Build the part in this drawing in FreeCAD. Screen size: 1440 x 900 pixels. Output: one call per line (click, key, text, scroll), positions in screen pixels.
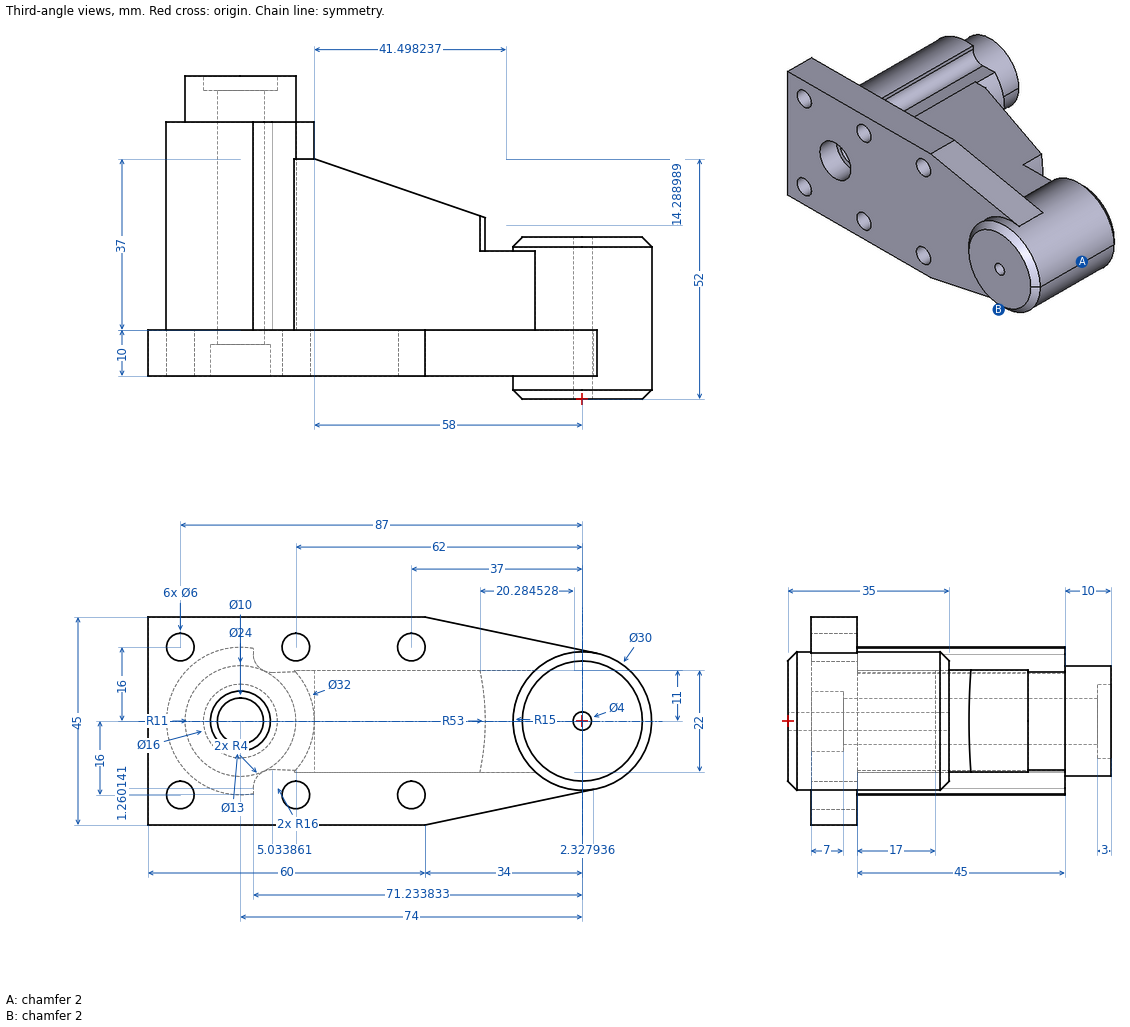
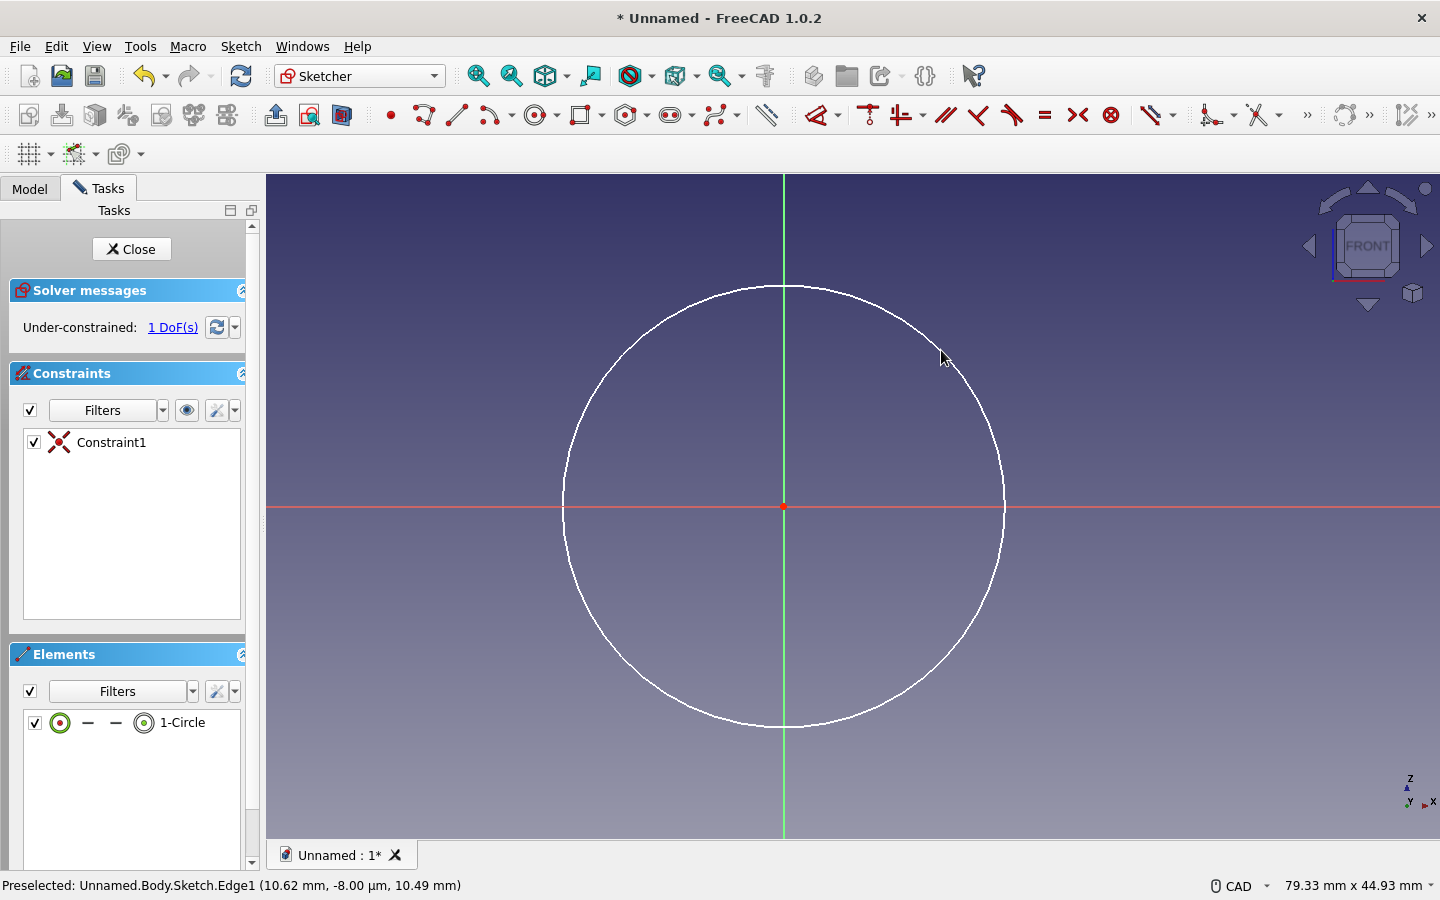
click(940, 350)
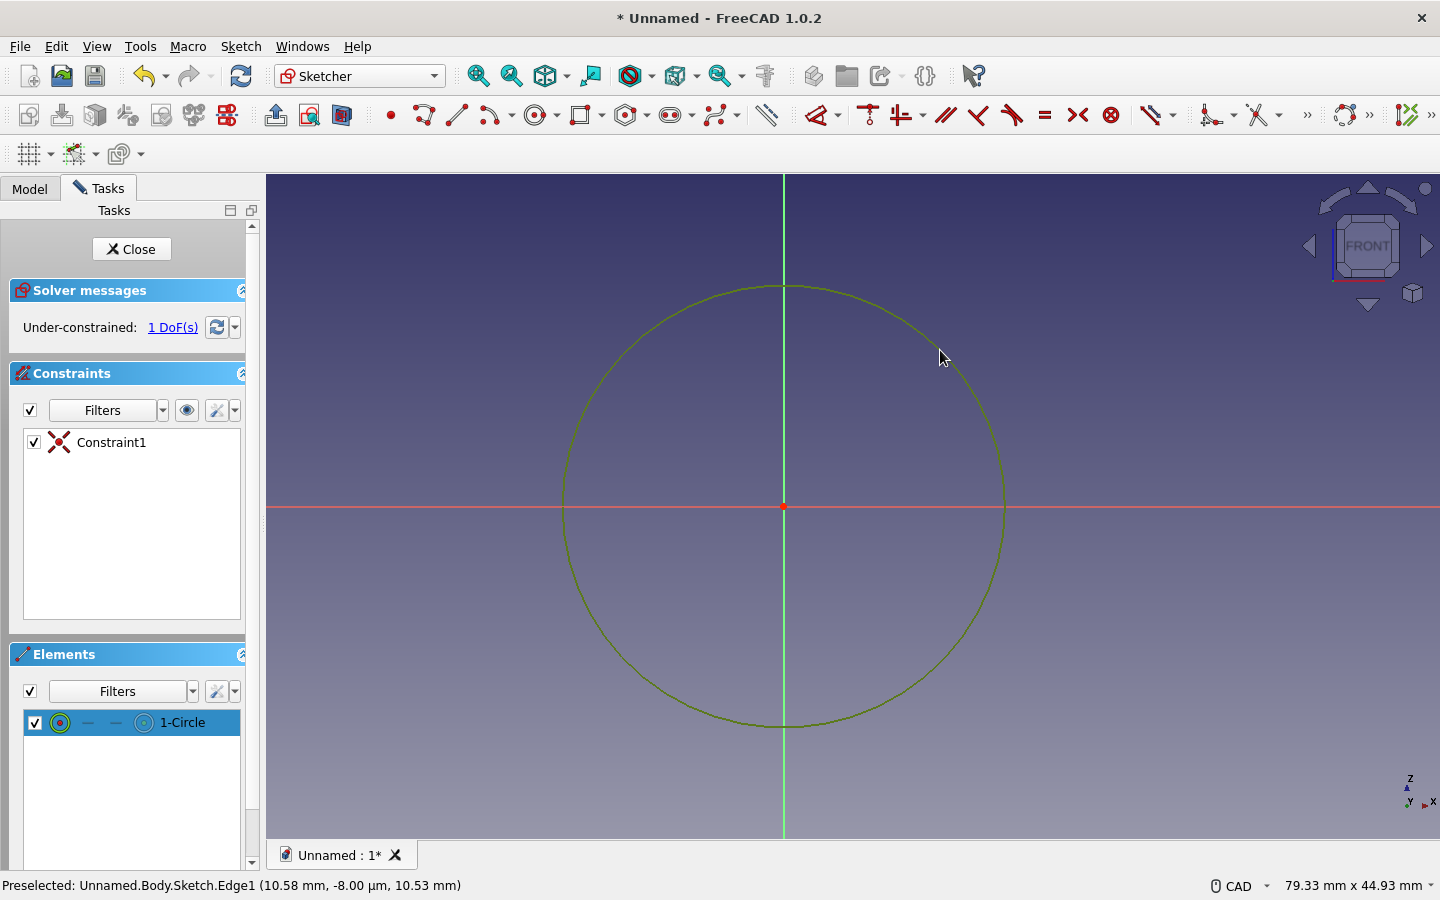
key(k)
key(o)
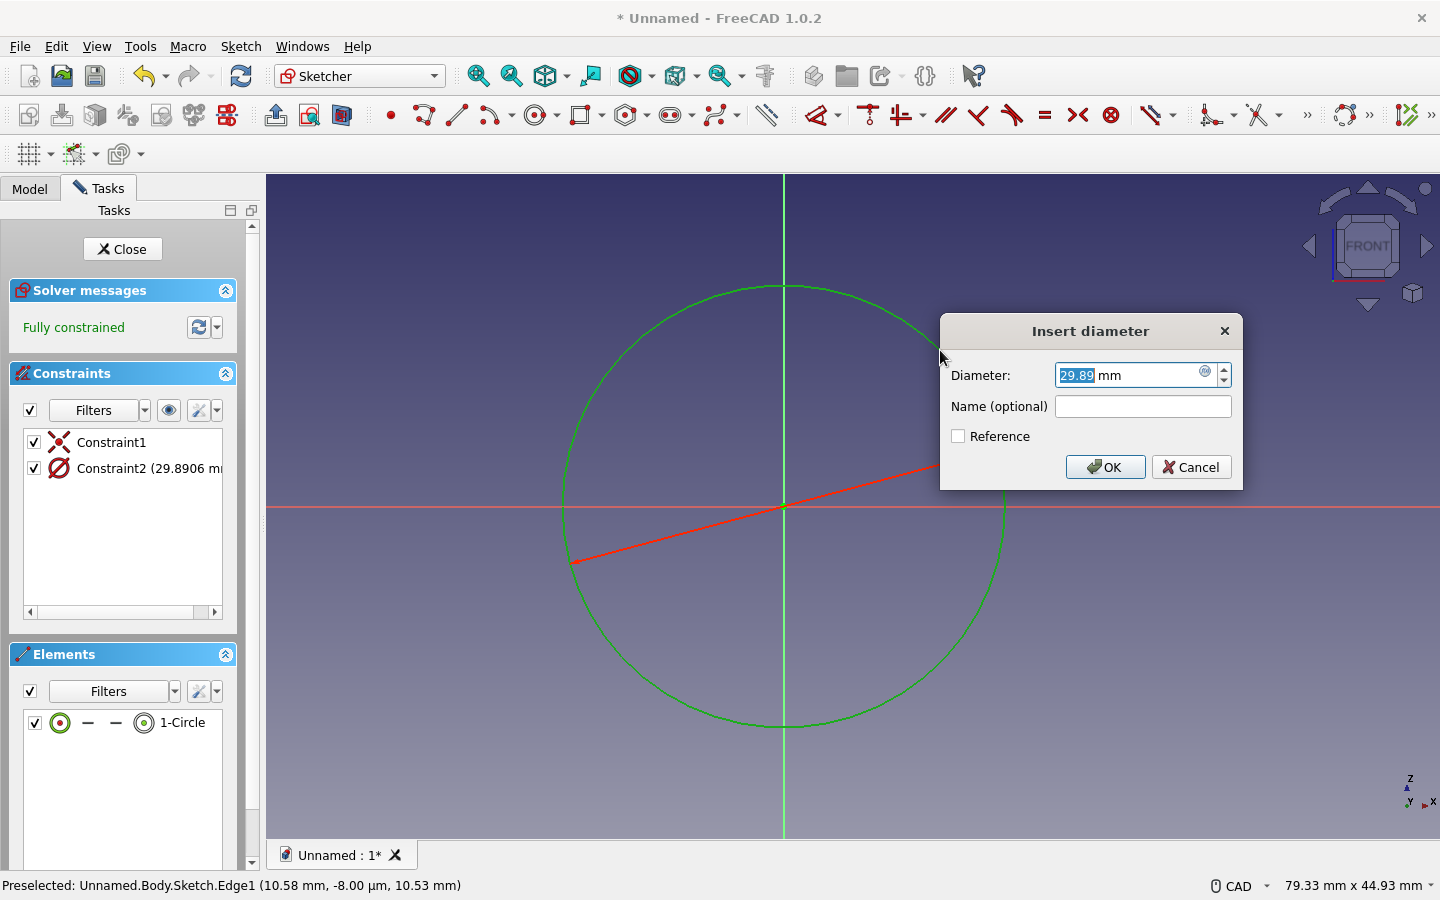
text(30)
key(Return)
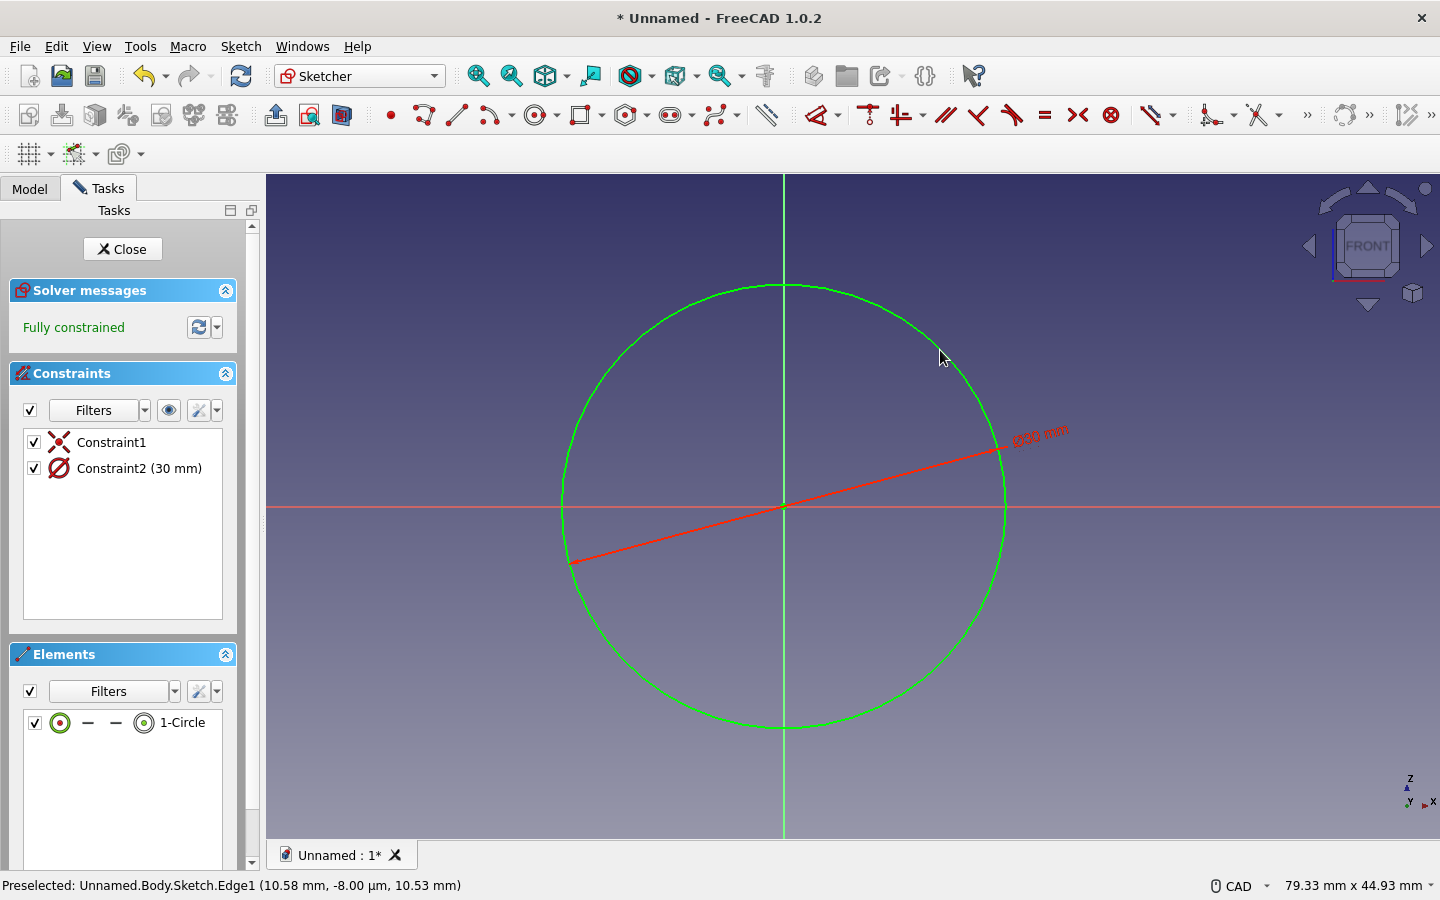
click(123, 249)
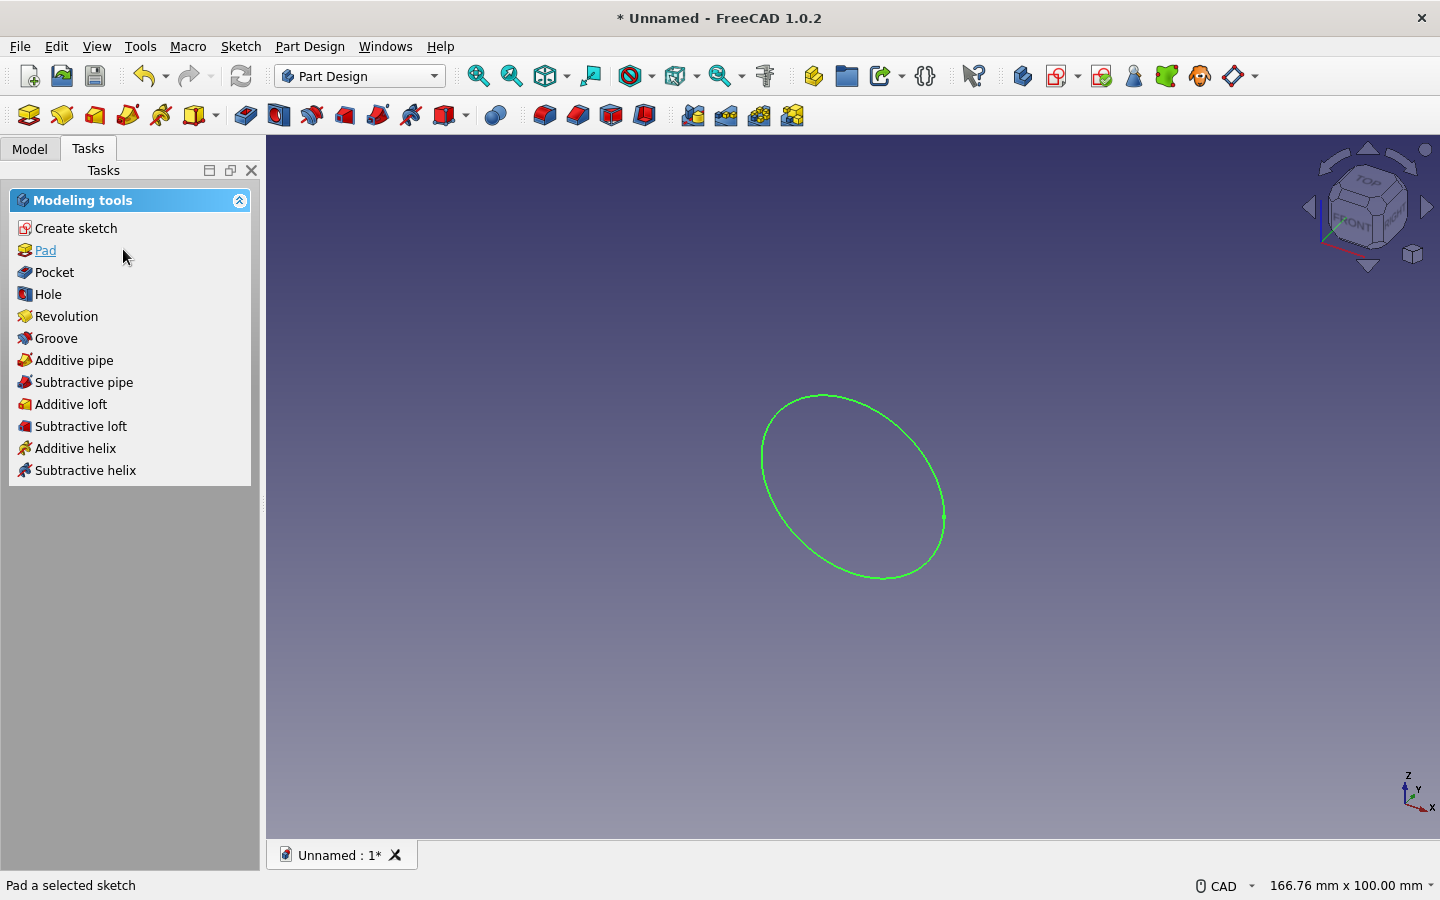
click(29, 116)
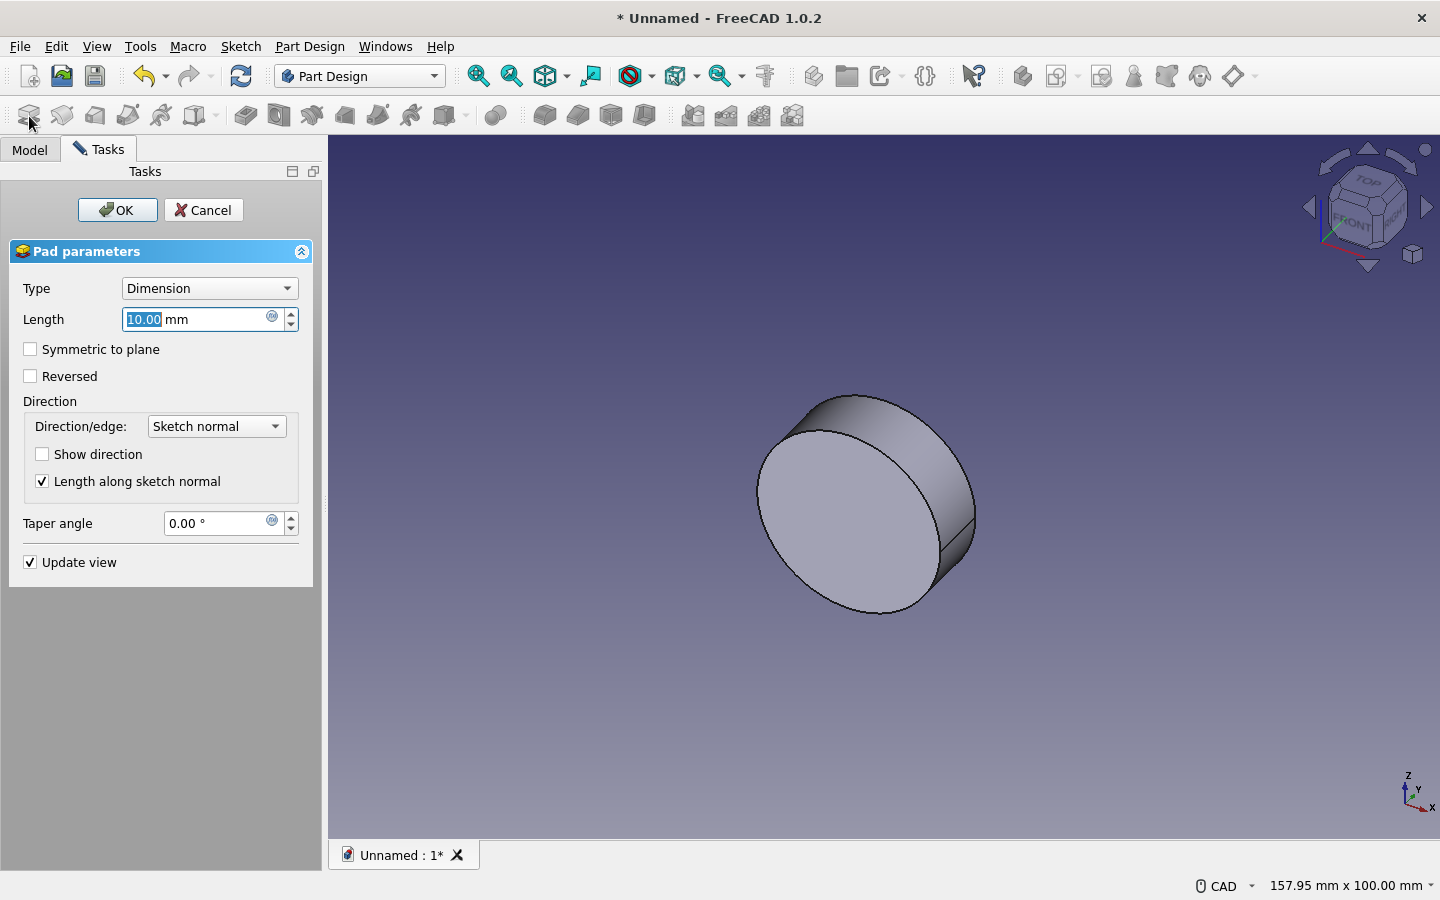
text(35)
key(Tab)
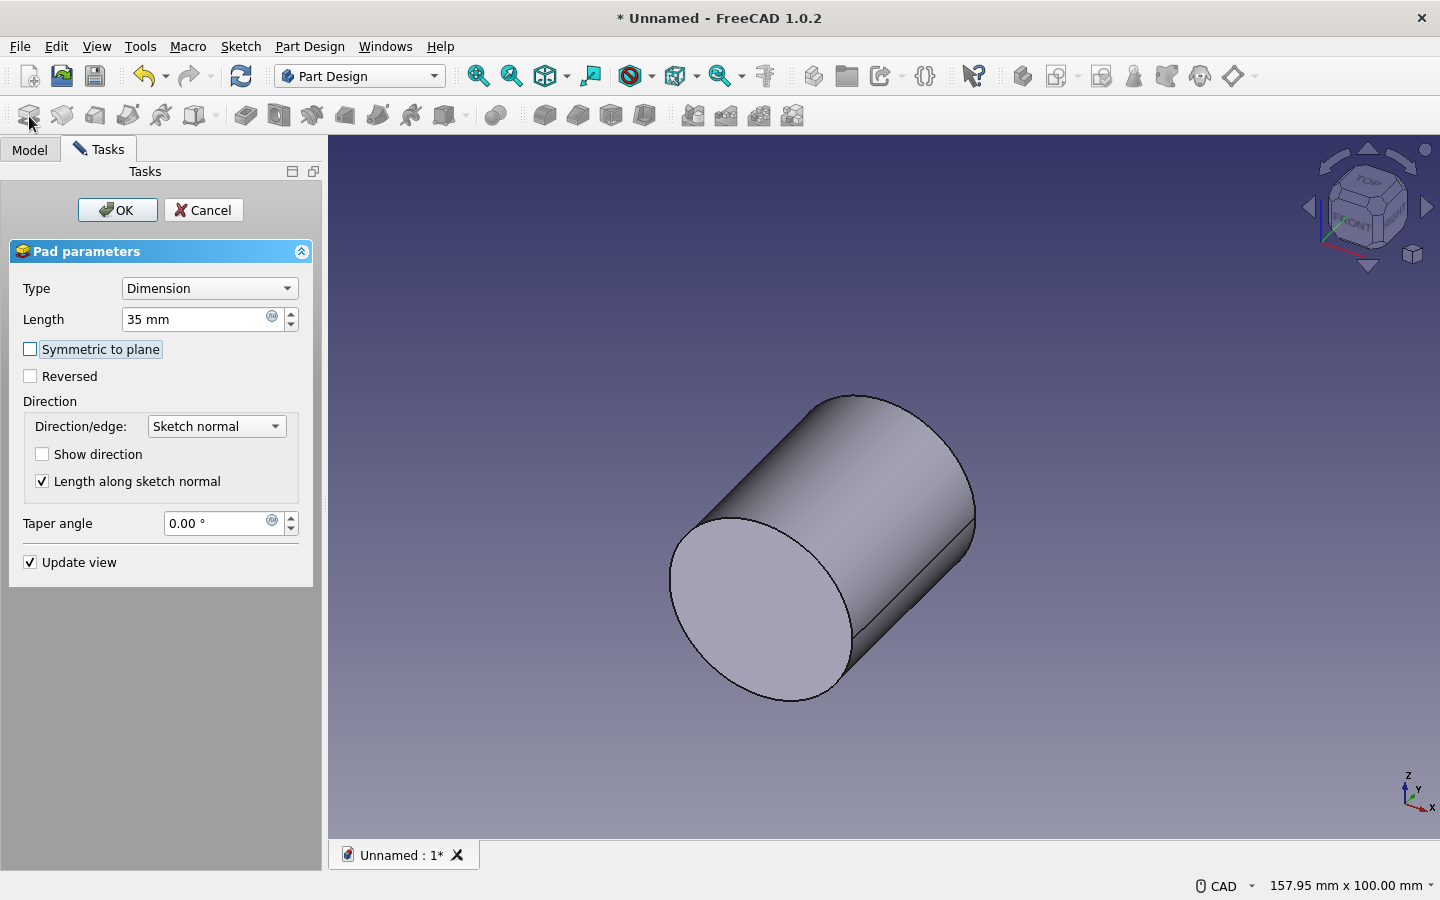
click(31, 376)